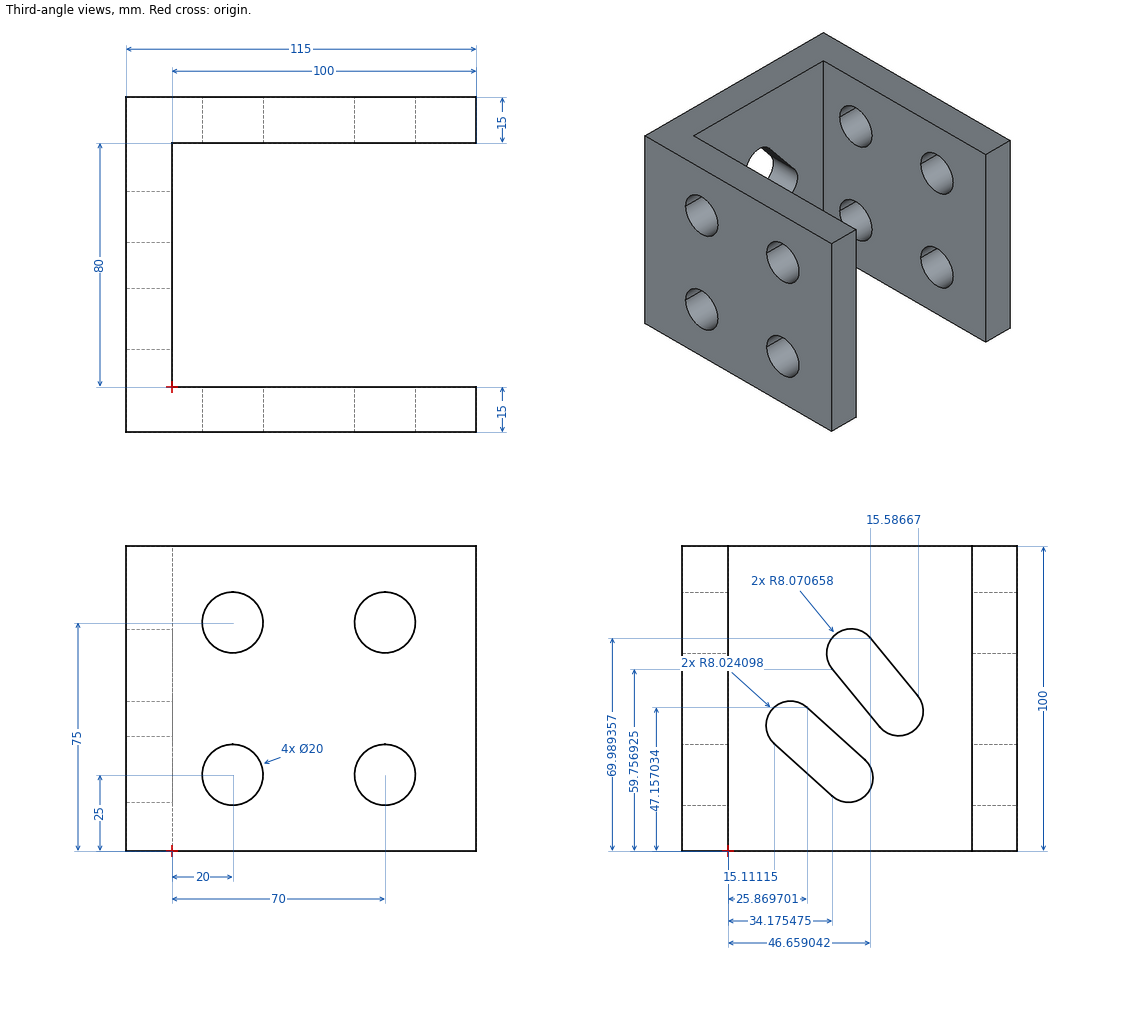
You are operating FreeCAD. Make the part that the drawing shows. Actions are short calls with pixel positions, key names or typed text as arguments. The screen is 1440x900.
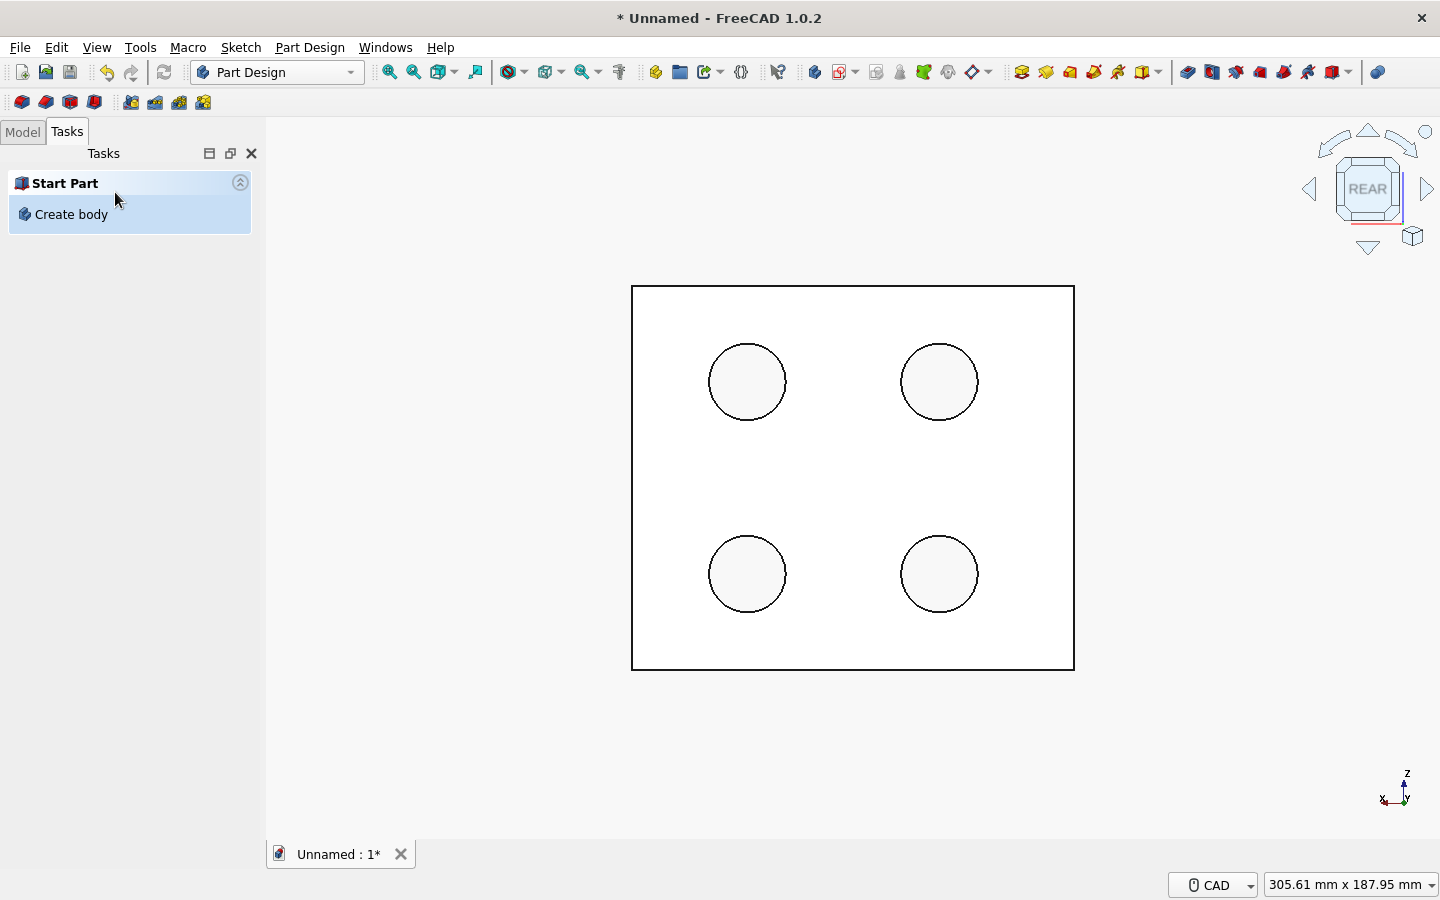
key(0)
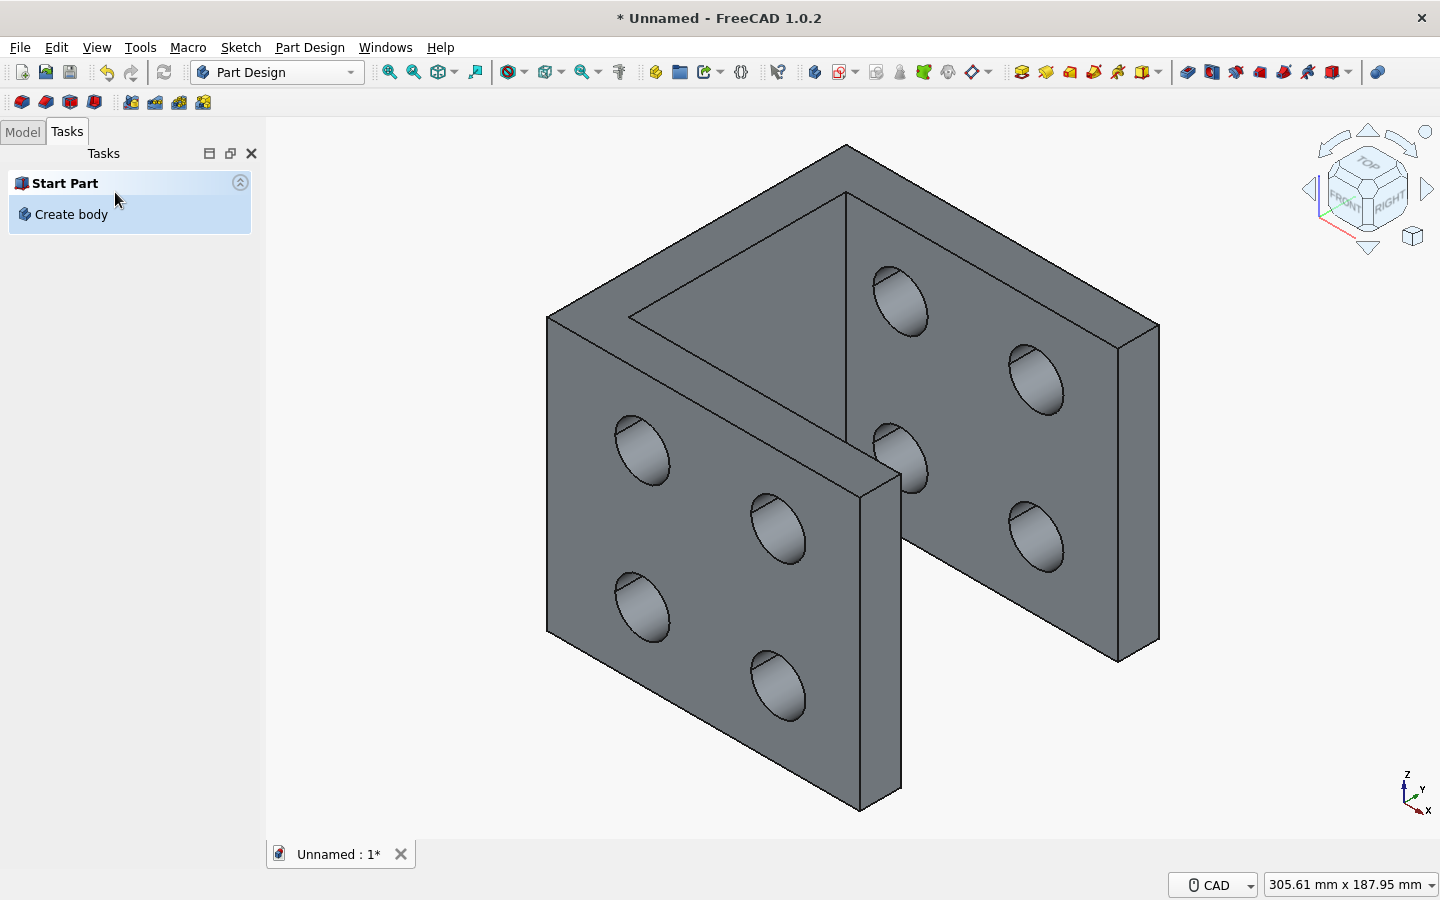
click(738, 366)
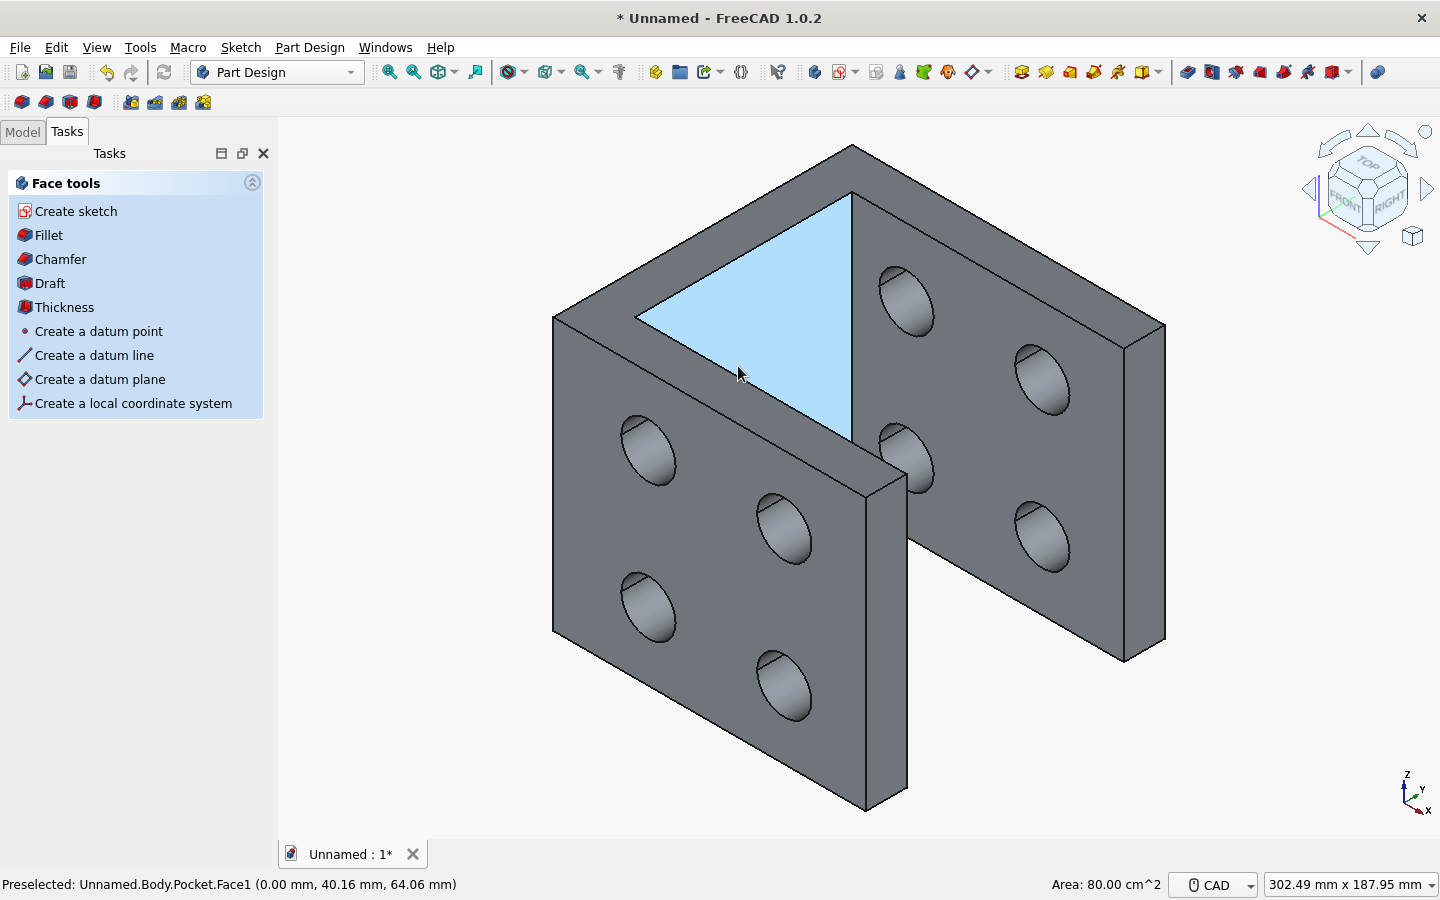
click(840, 72)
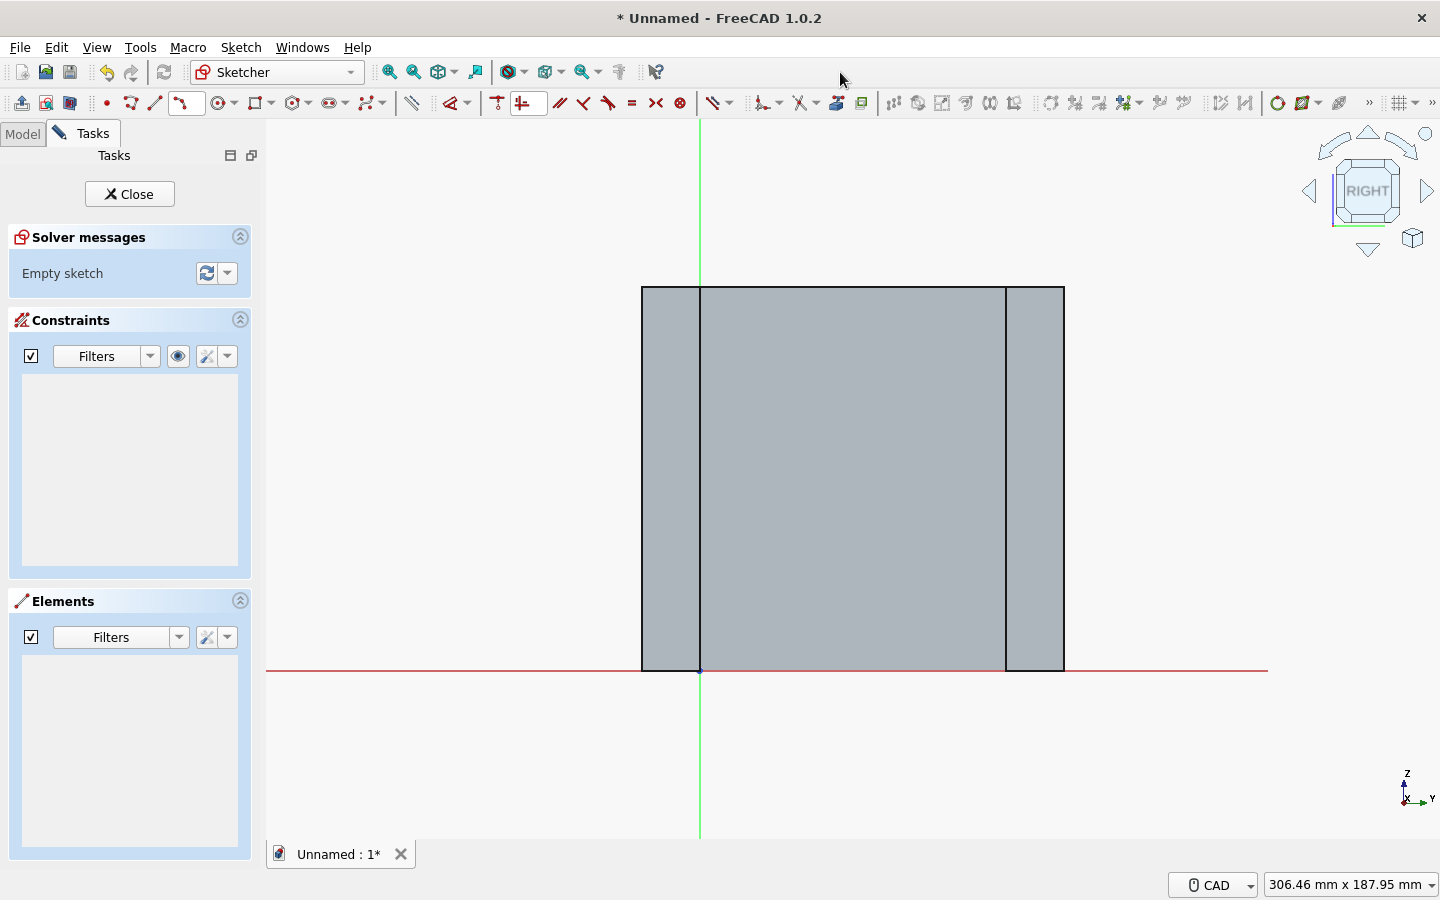
key(q)
key(s)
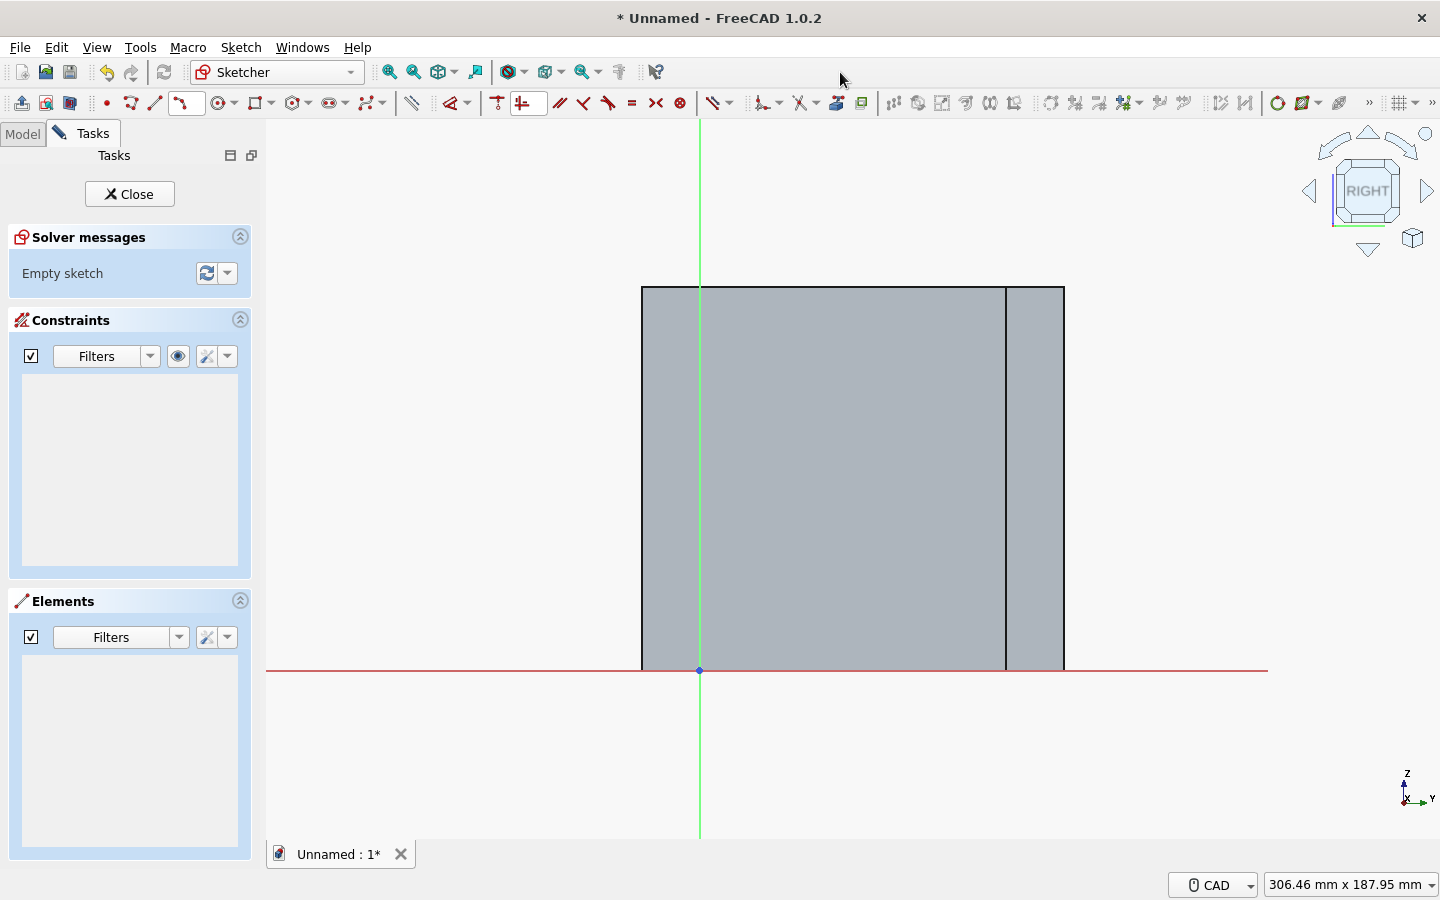
scroll(861, 602, up, 3)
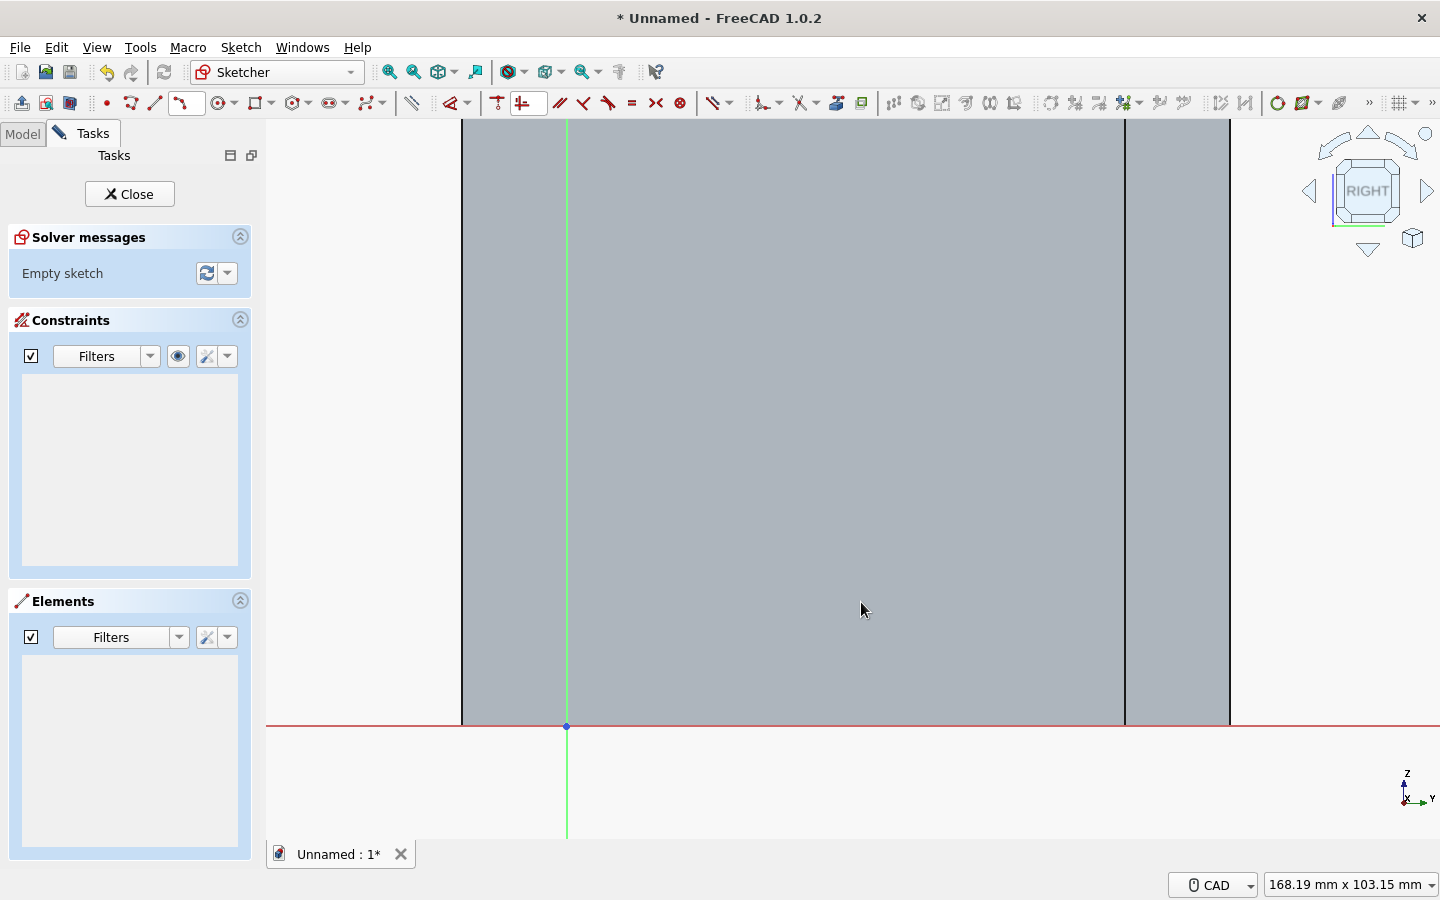
key(g)
key(s)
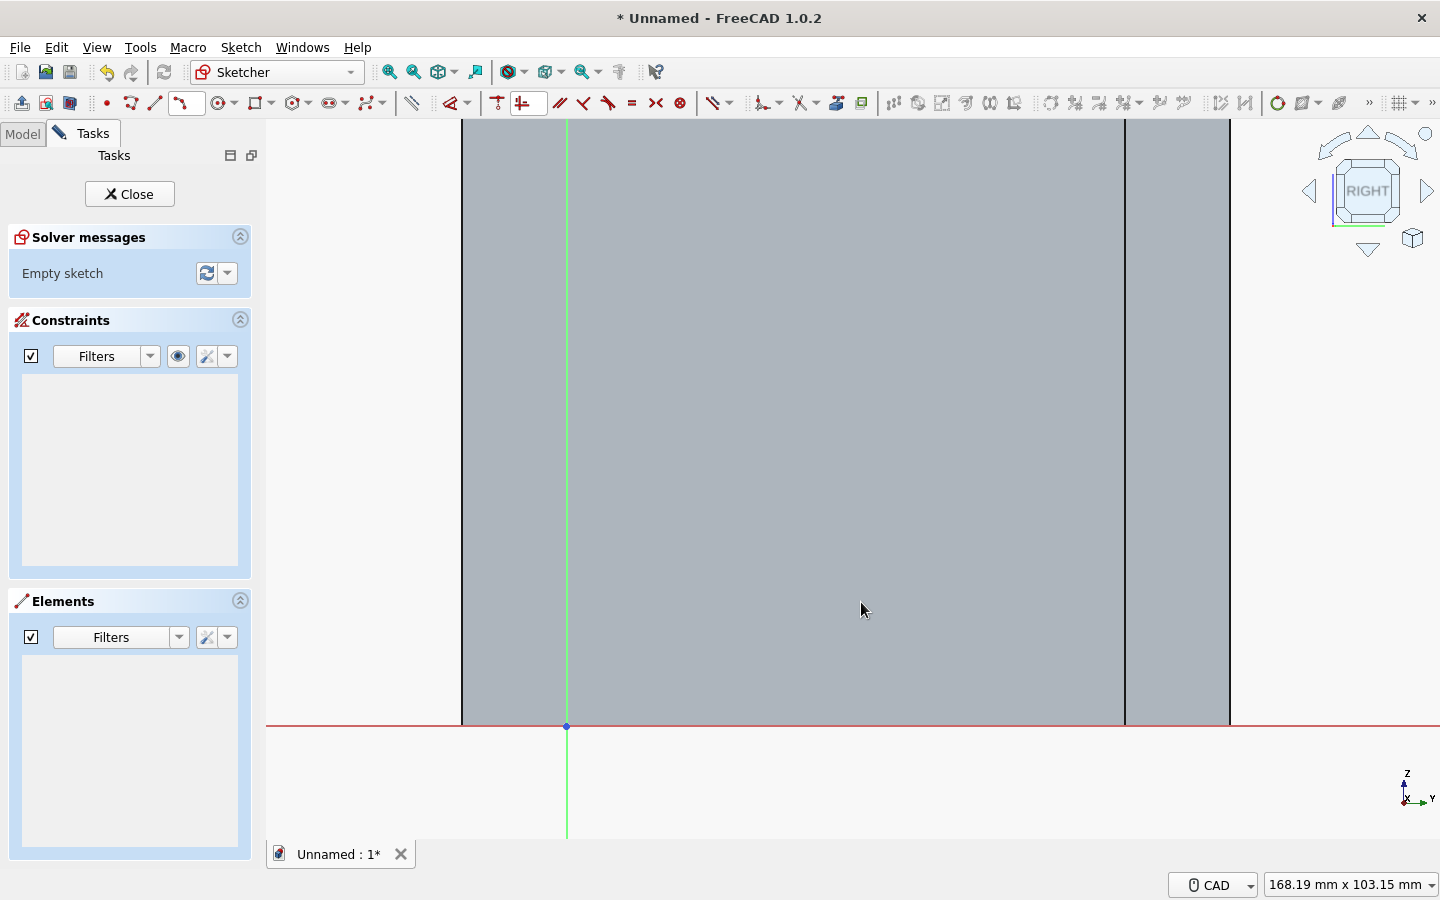
click(849, 274)